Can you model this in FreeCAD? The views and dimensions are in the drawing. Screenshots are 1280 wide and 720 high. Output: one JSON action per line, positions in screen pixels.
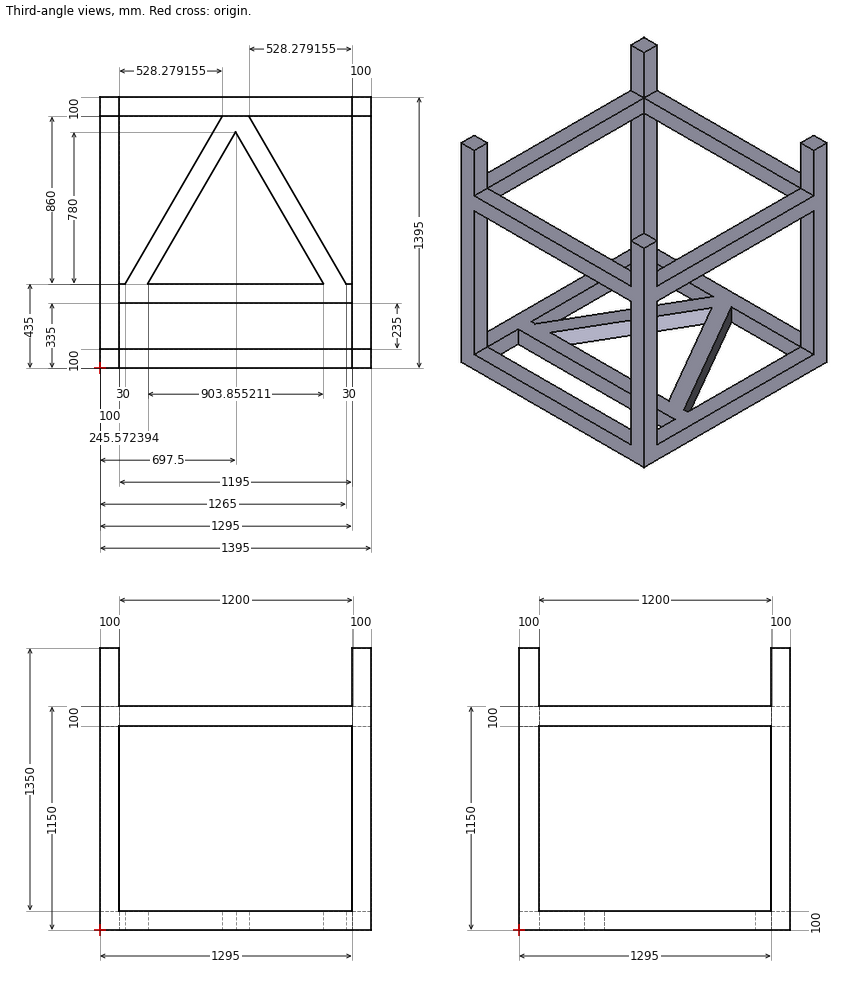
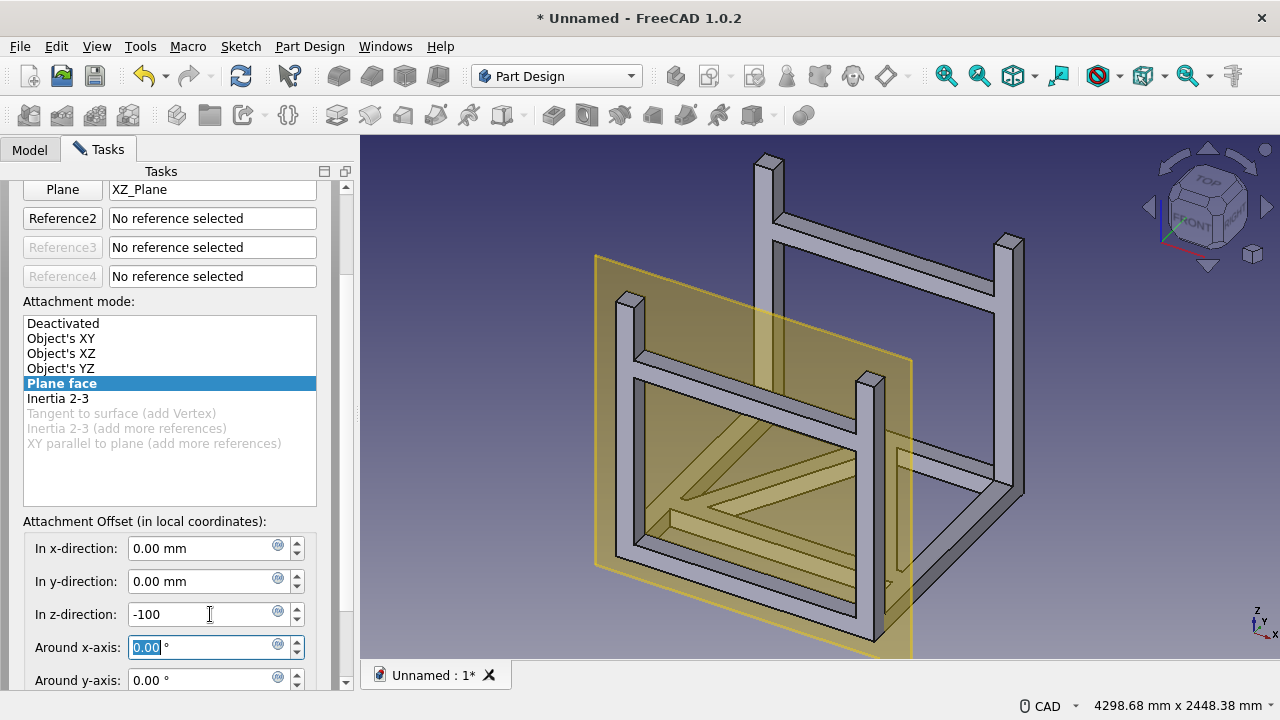
{"action": "scroll", "coordinate": [346, 436], "scroll_direction": "up", "scroll_amount": 3}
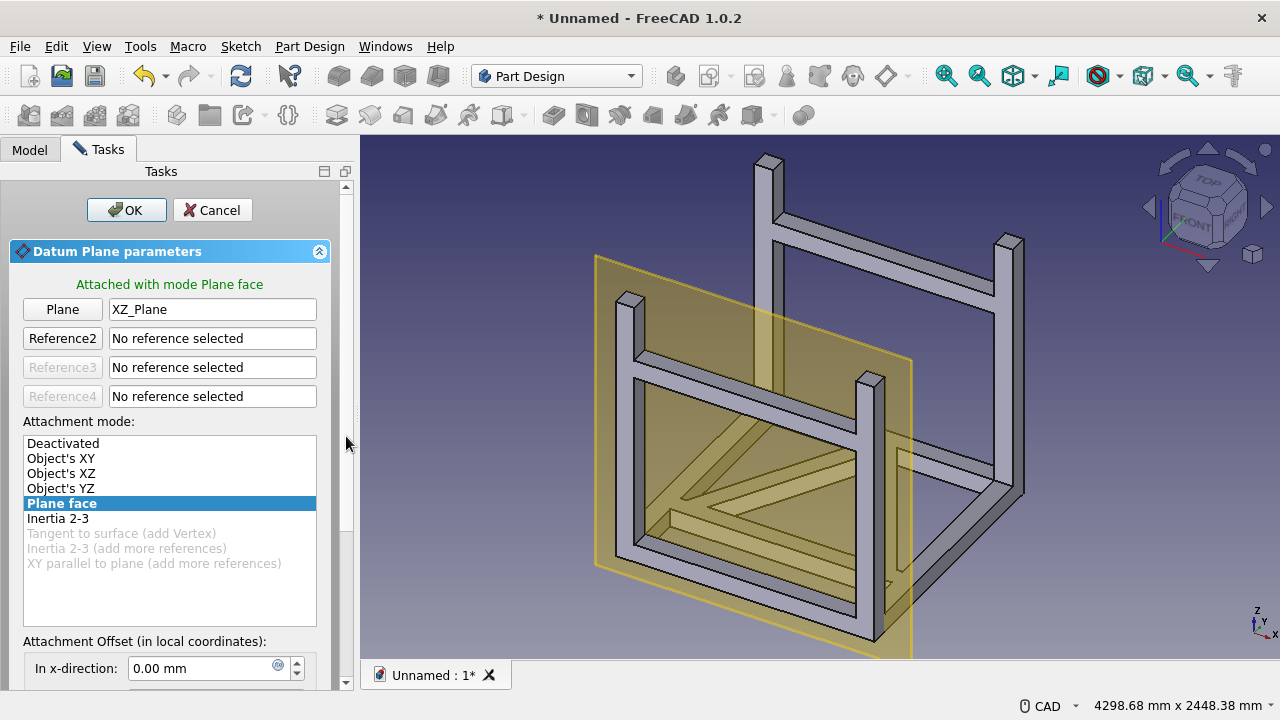
{"action": "left_click", "coordinate": [127, 210]}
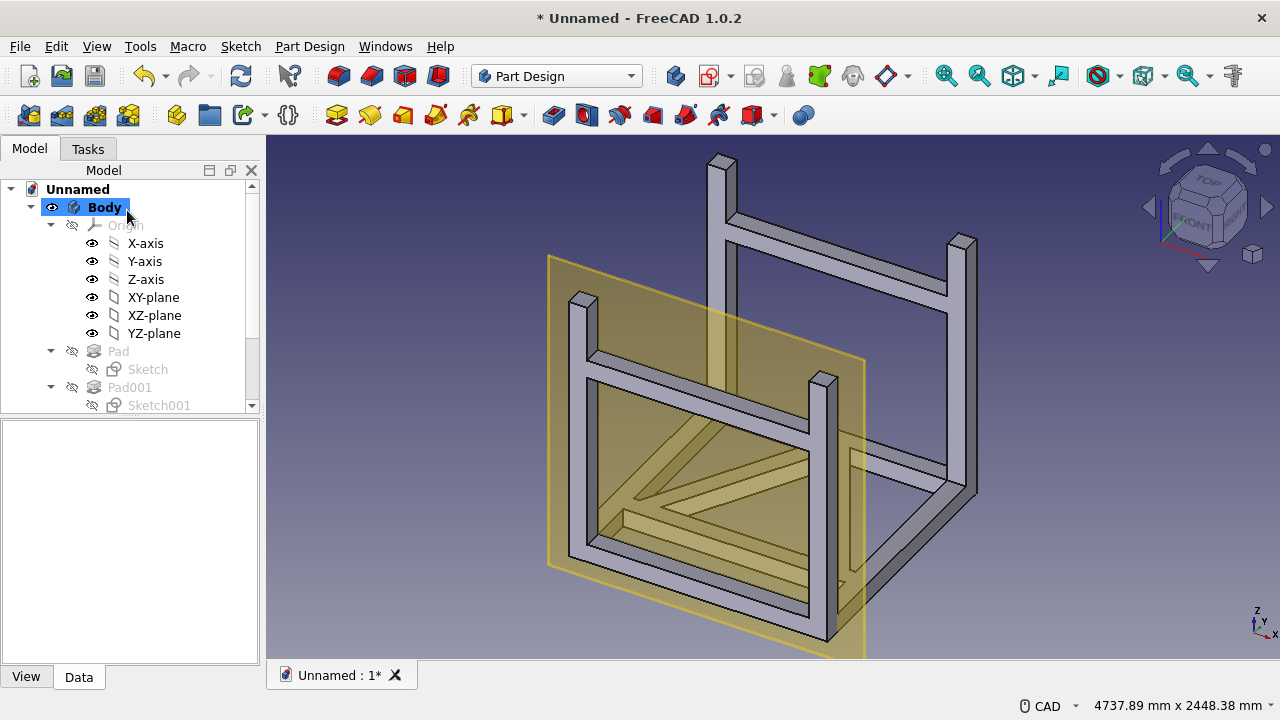
{"action": "scroll", "coordinate": [101, 293], "scroll_direction": "down", "scroll_amount": 3}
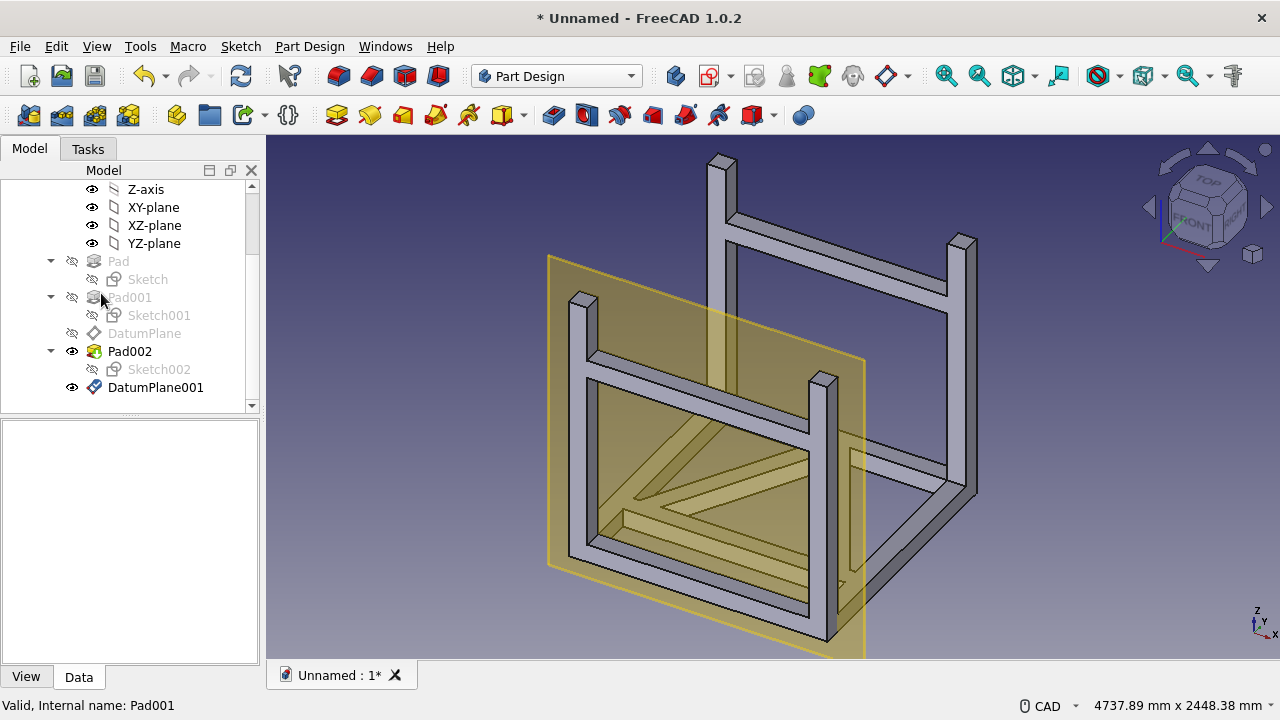
{"action": "left_click", "coordinate": [117, 387]}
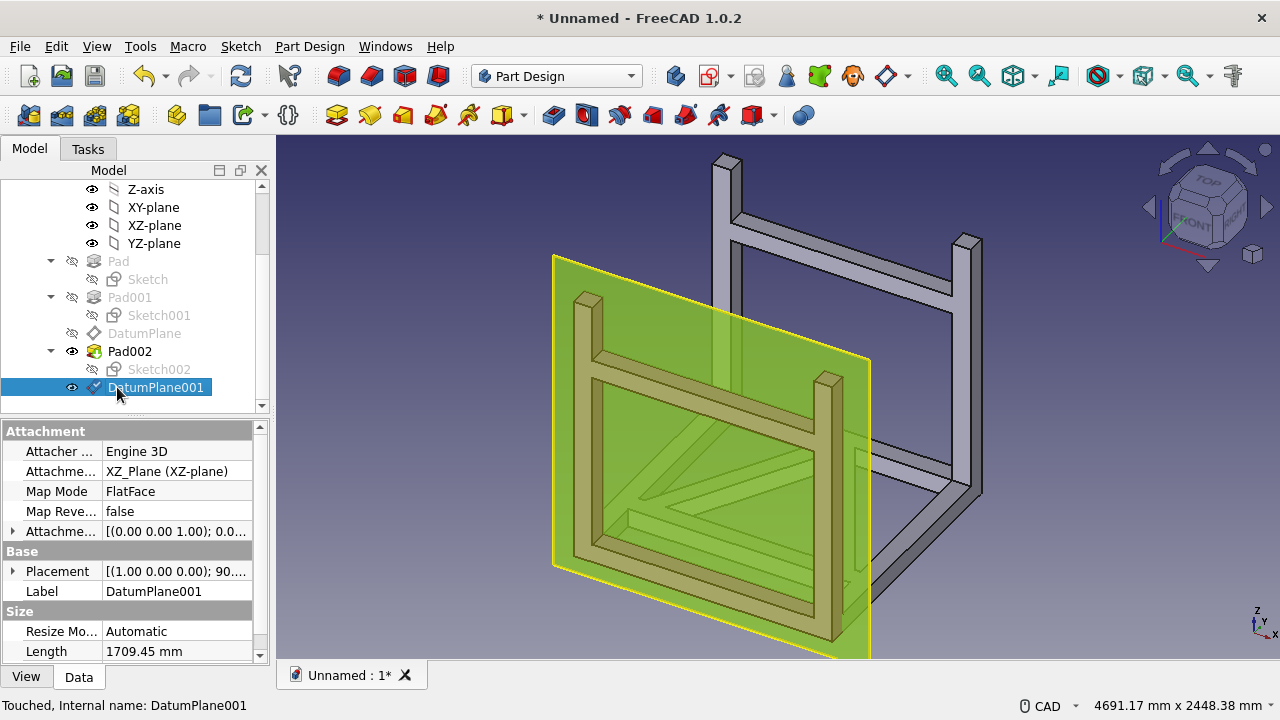
{"action": "left_click", "coordinate": [708, 76]}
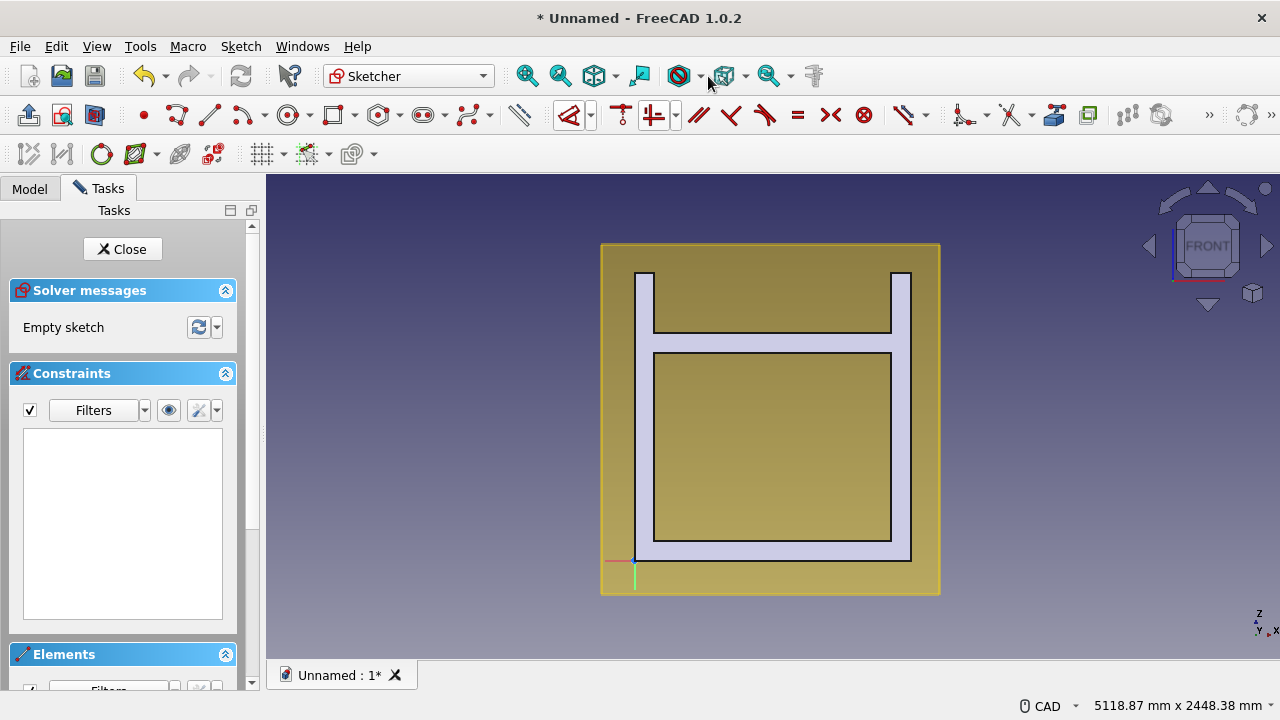
{"action": "left_click", "coordinate": [95, 116]}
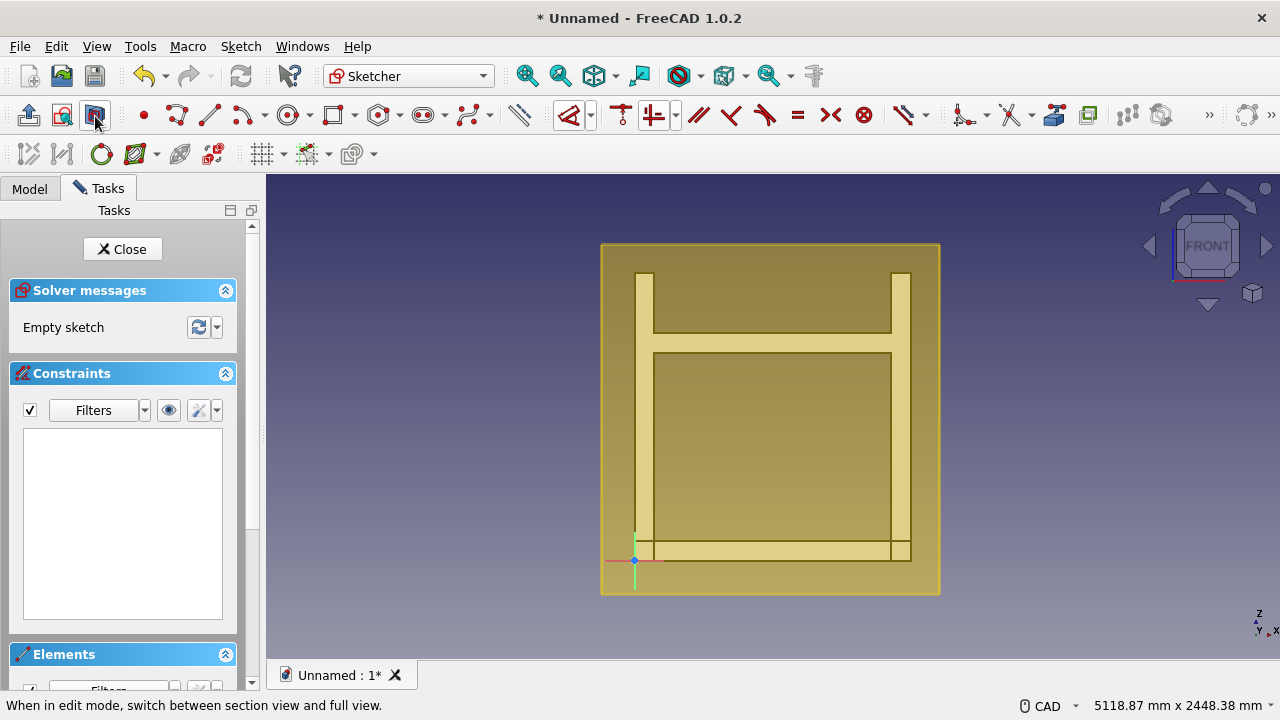
{"action": "left_click", "coordinate": [332, 116]}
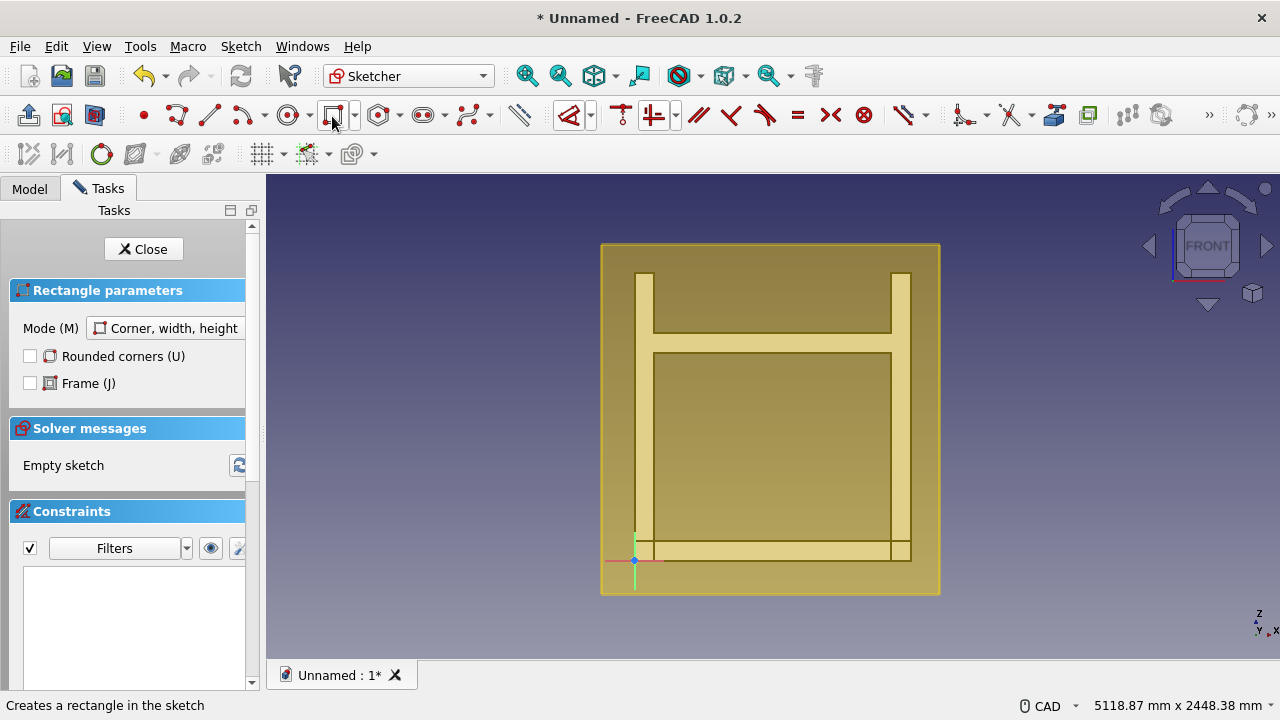
{"action": "left_click", "coordinate": [635, 333]}
{"action": "mouse_move", "coordinate": [654, 353]}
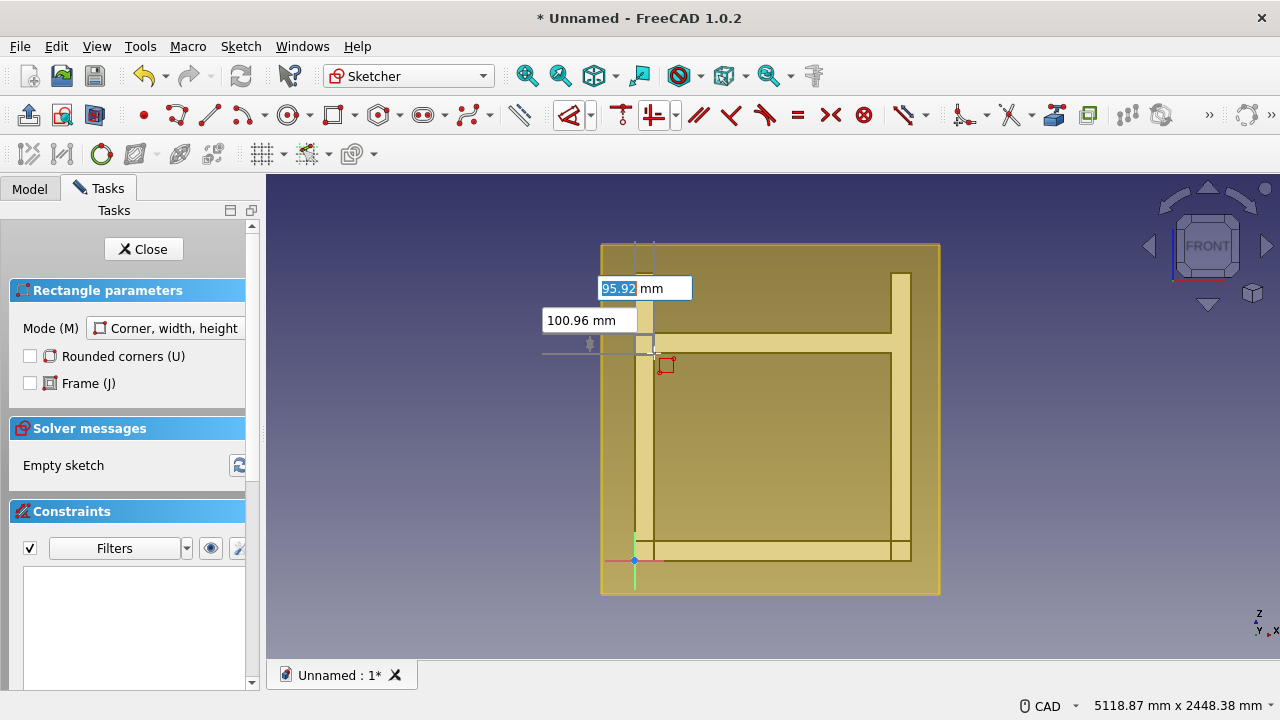
{"action": "type", "text": "100"}
{"action": "key", "text": "Tab"}
{"action": "type", "text": "100"}
{"action": "key", "text": "Return"}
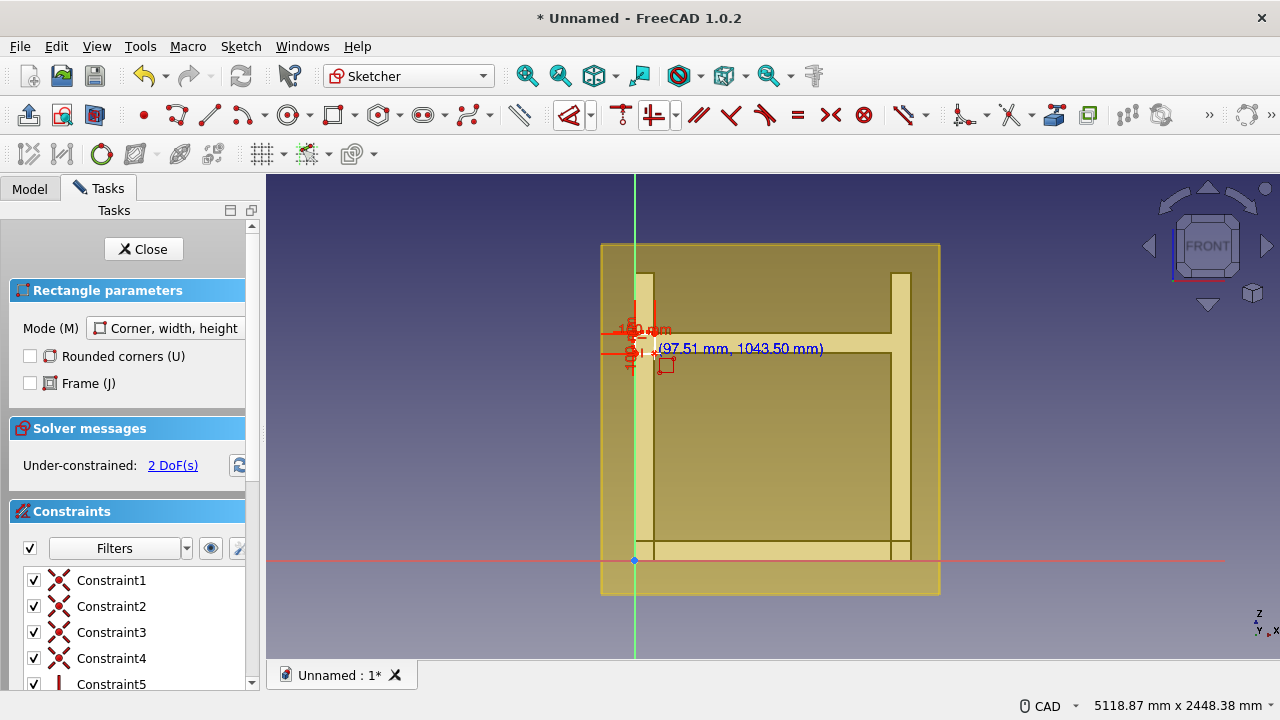
{"action": "left_click", "coordinate": [891, 333]}
{"action": "mouse_move", "coordinate": [911, 353]}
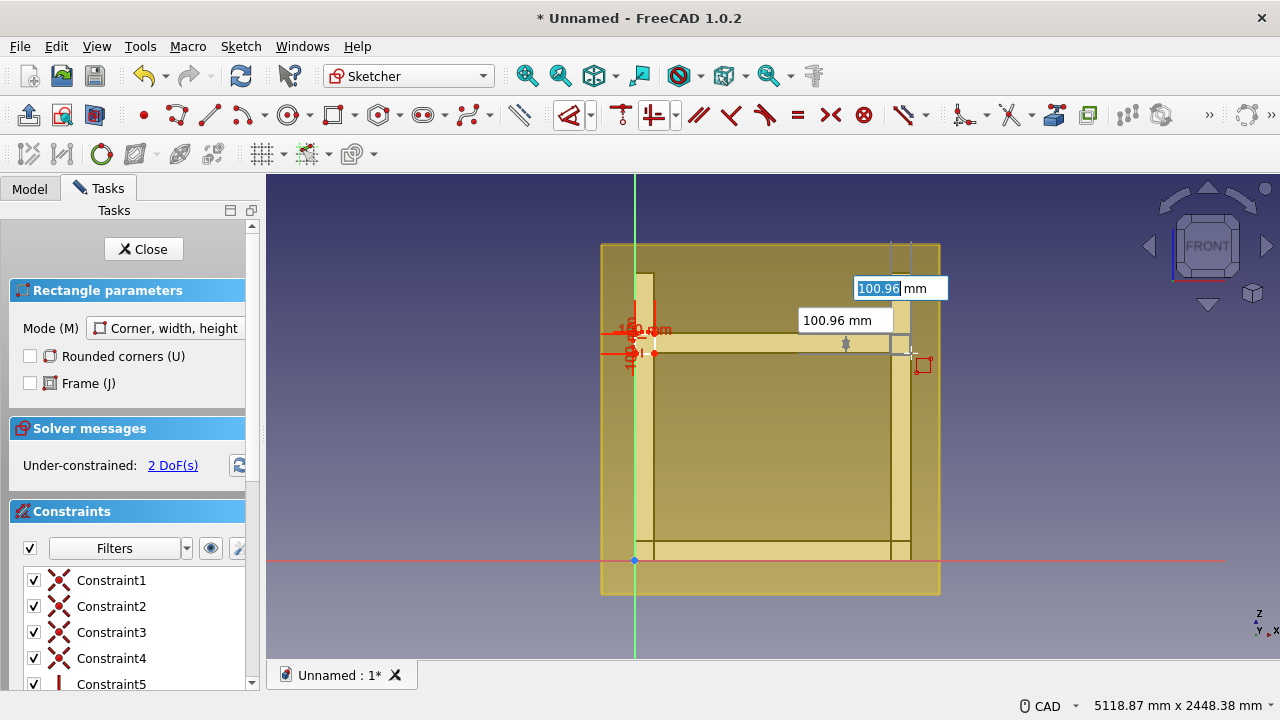
{"action": "type", "text": "100"}
{"action": "key", "text": "Tab"}
{"action": "type", "text": "100"}
{"action": "key", "text": "Return"}
{"action": "key", "text": "Escape"}